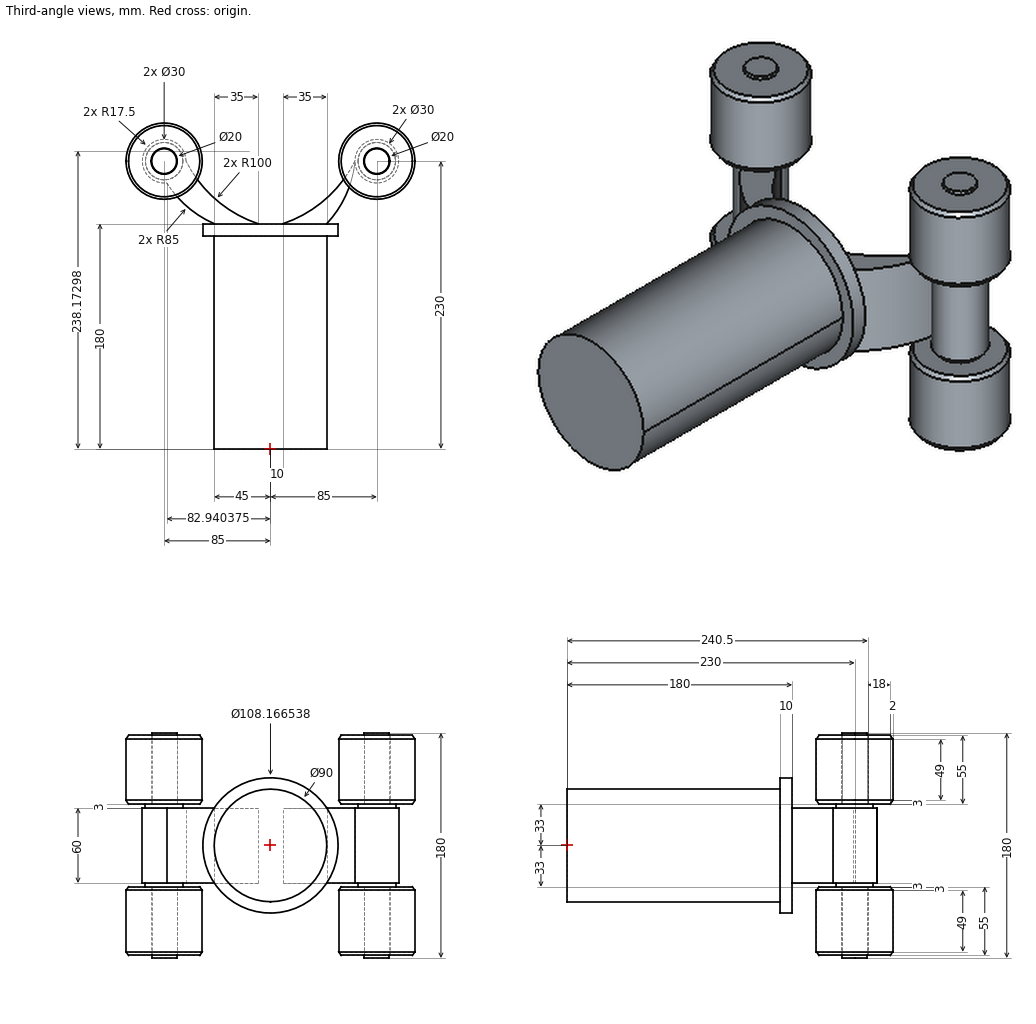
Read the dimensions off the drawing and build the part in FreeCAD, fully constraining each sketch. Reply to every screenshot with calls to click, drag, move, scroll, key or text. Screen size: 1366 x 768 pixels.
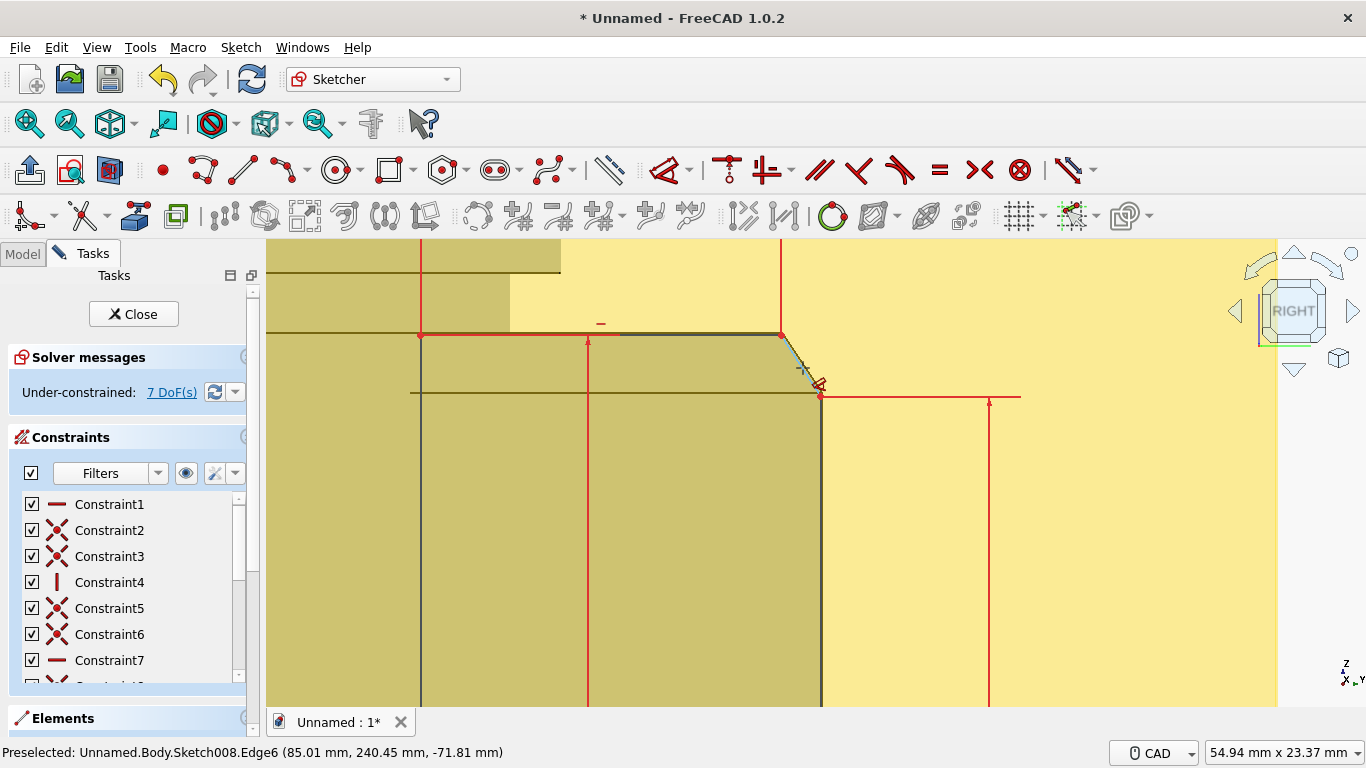
click(801, 366)
click(801, 301)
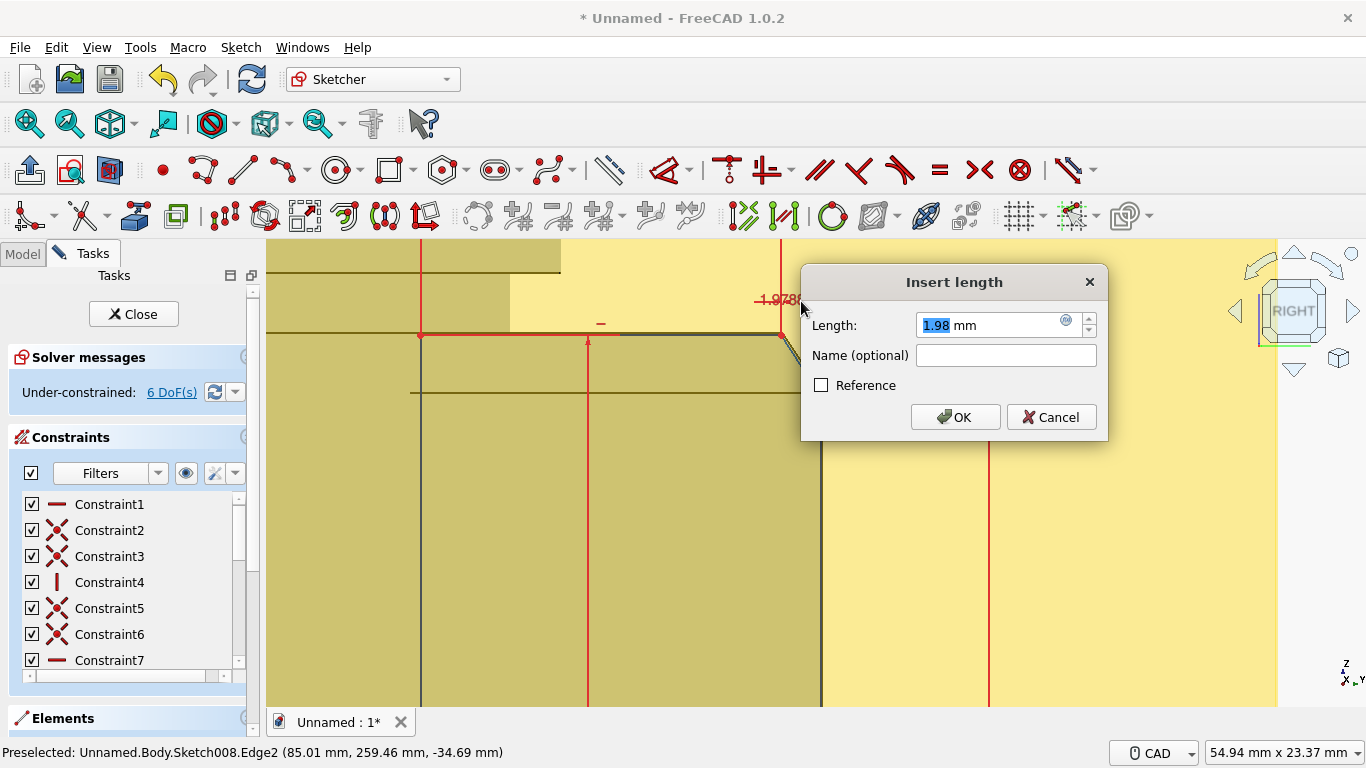
text(2)
key(Return)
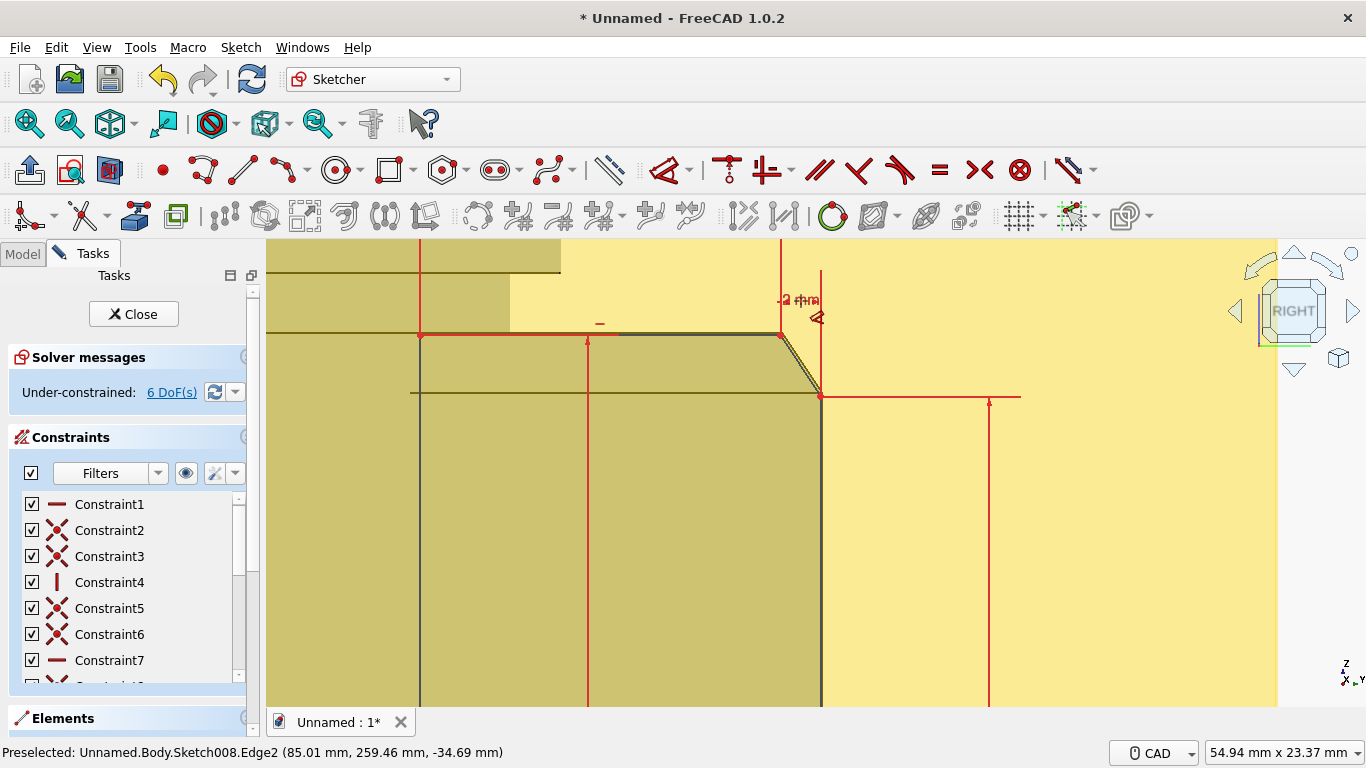
click(793, 354)
click(855, 366)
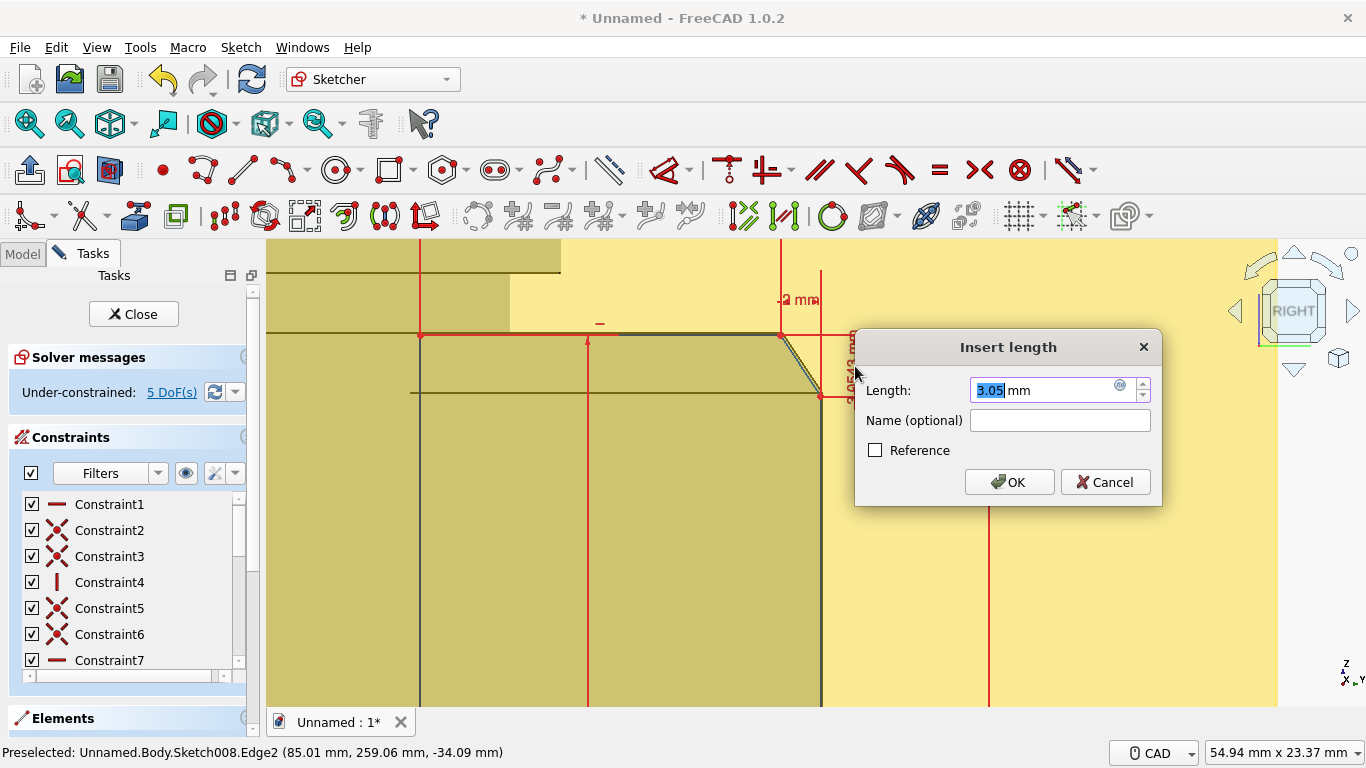
text(3)
key(Return)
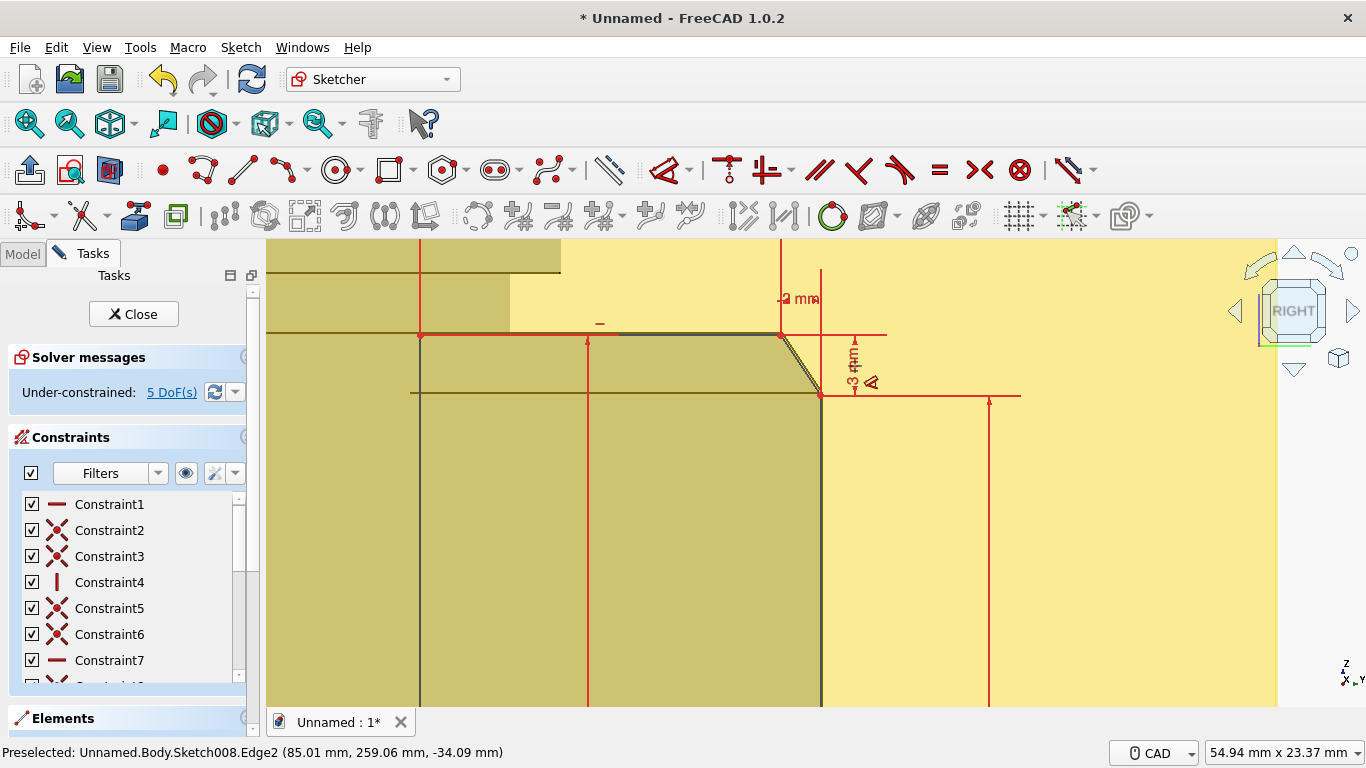
scroll(806, 369, down, 8)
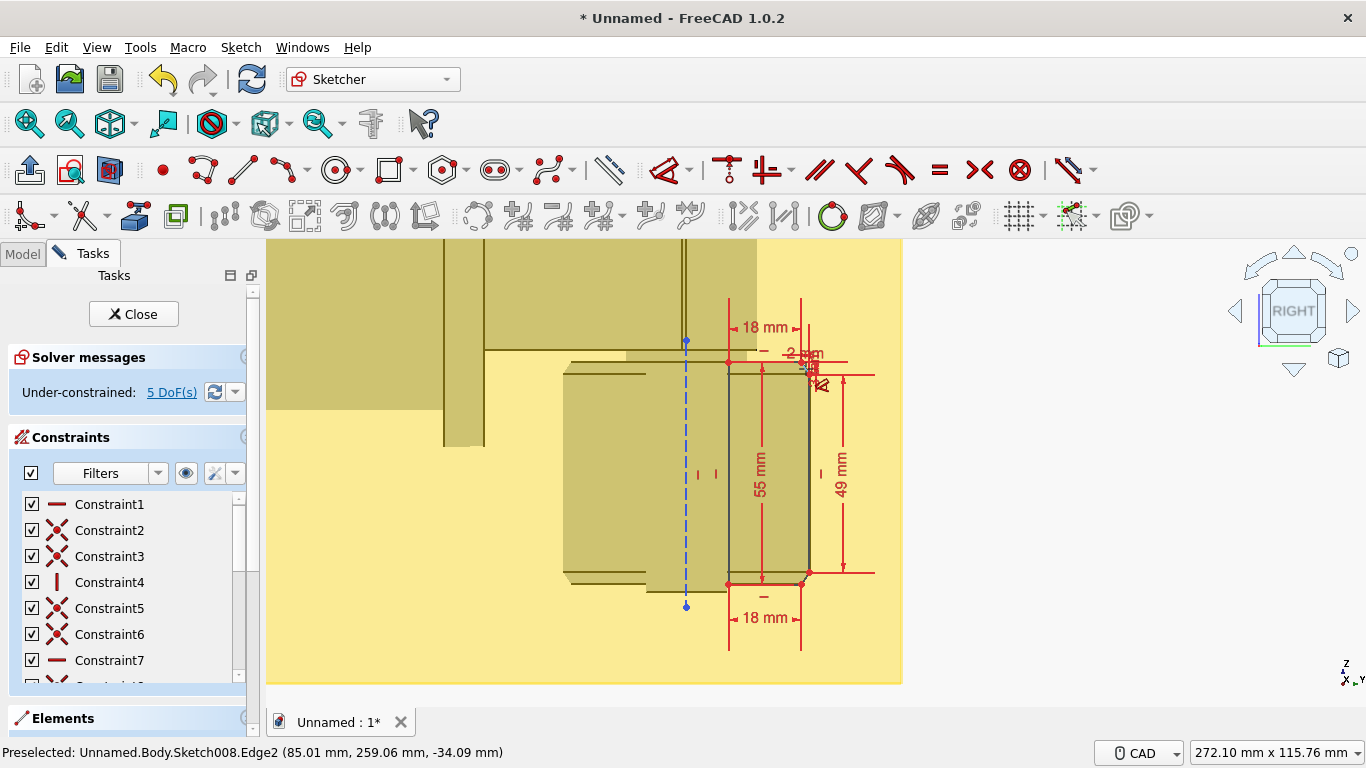
click(729, 362)
click(763, 293)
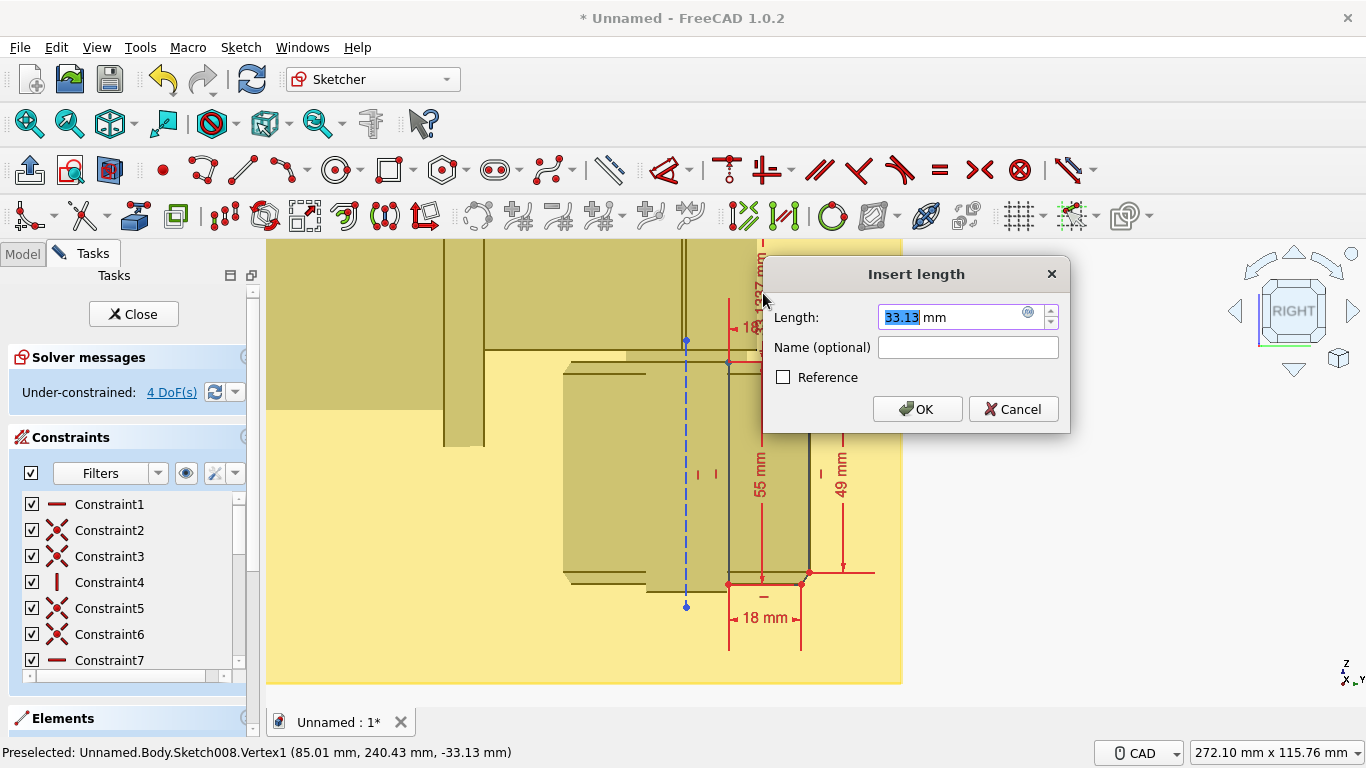
text(33)
key(Return)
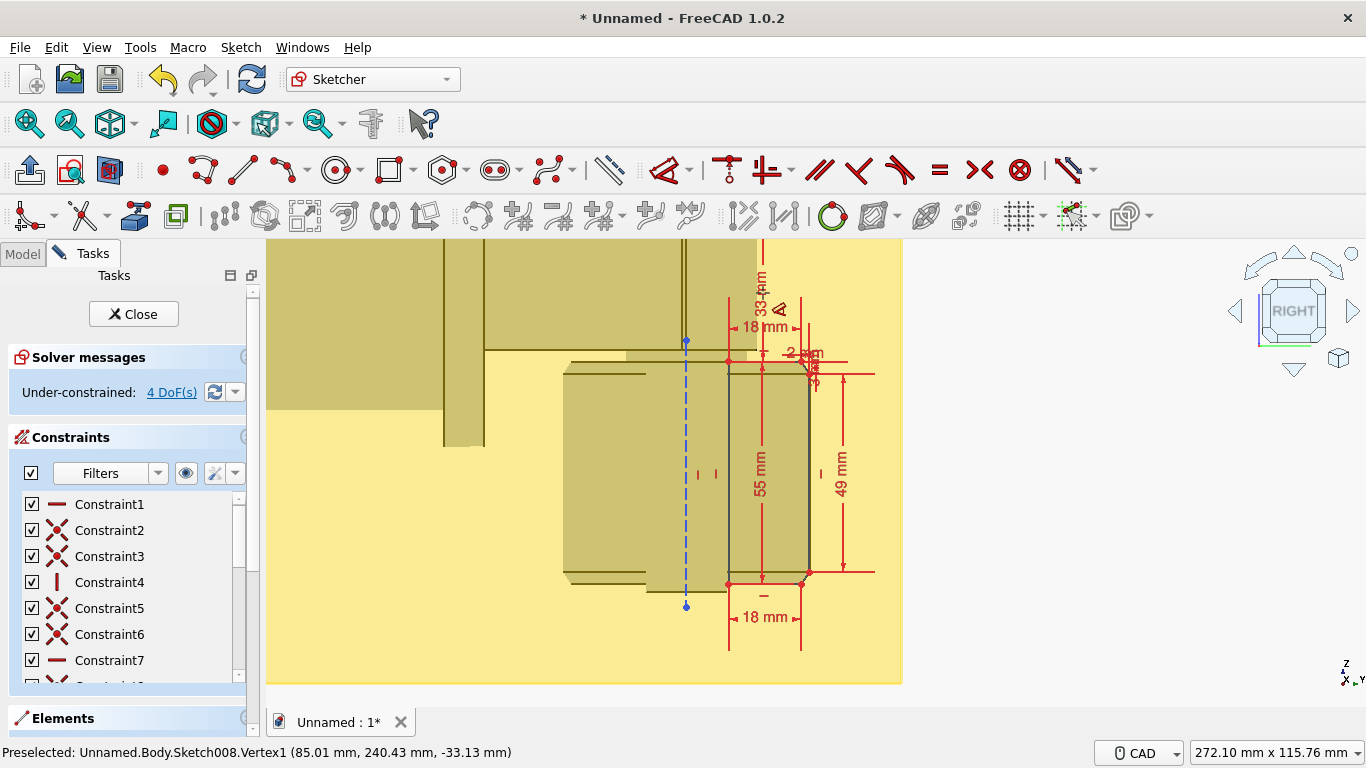
click(686, 341)
click(490, 375)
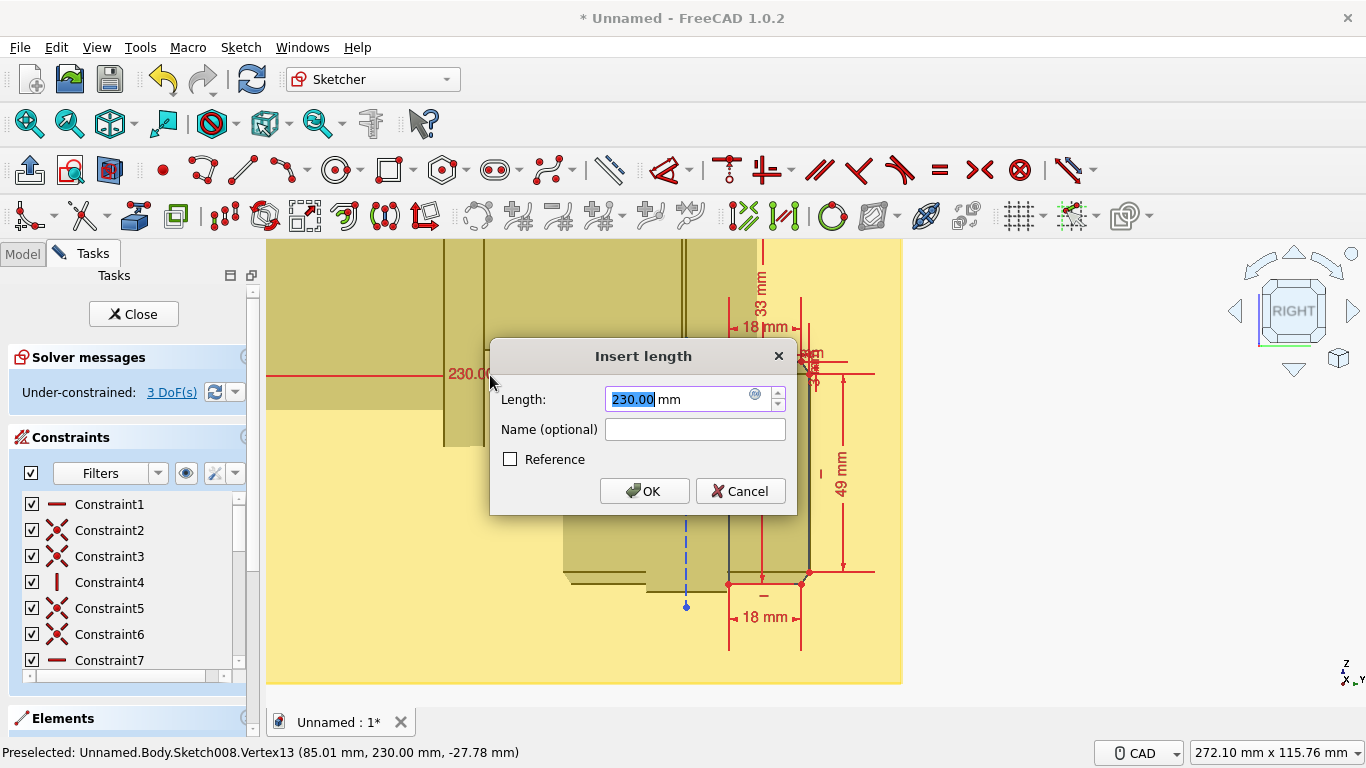
text(230)
key(Return)